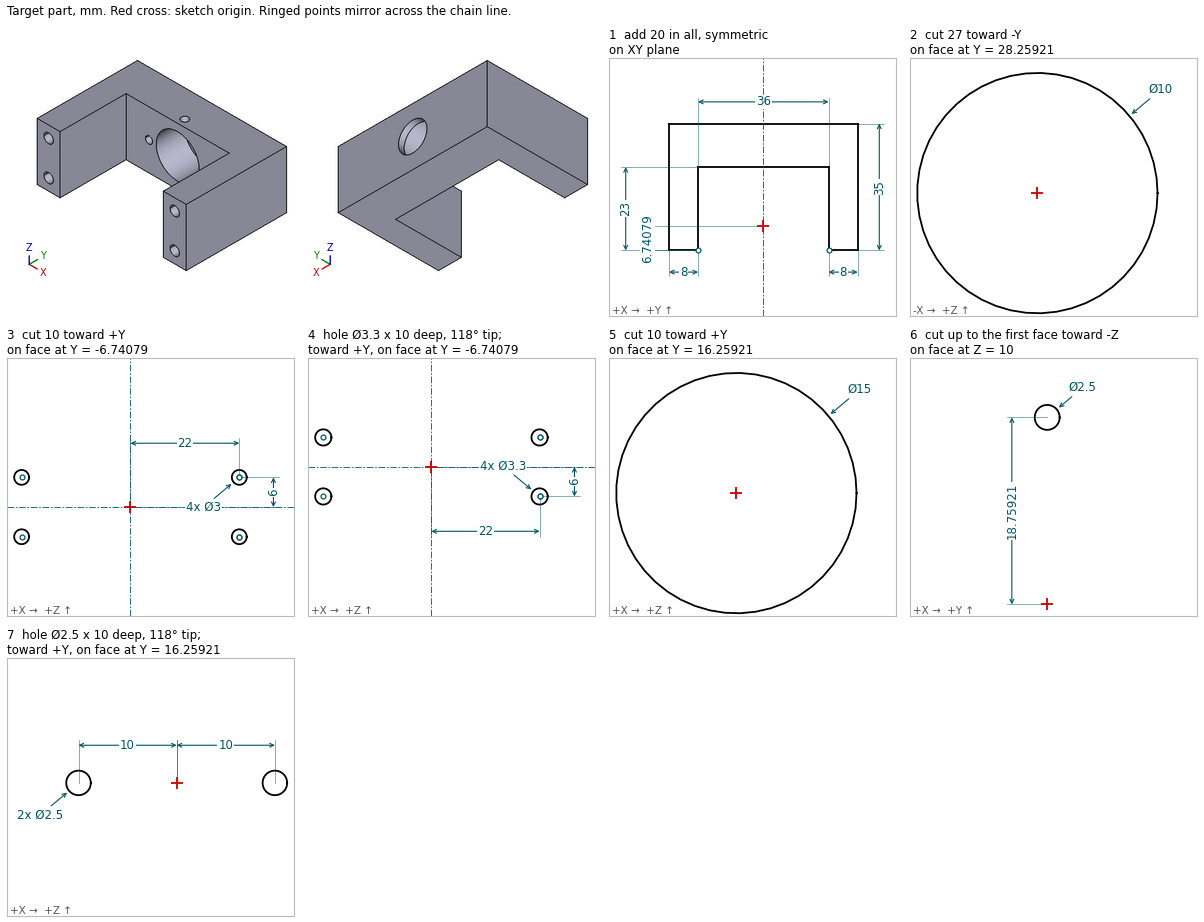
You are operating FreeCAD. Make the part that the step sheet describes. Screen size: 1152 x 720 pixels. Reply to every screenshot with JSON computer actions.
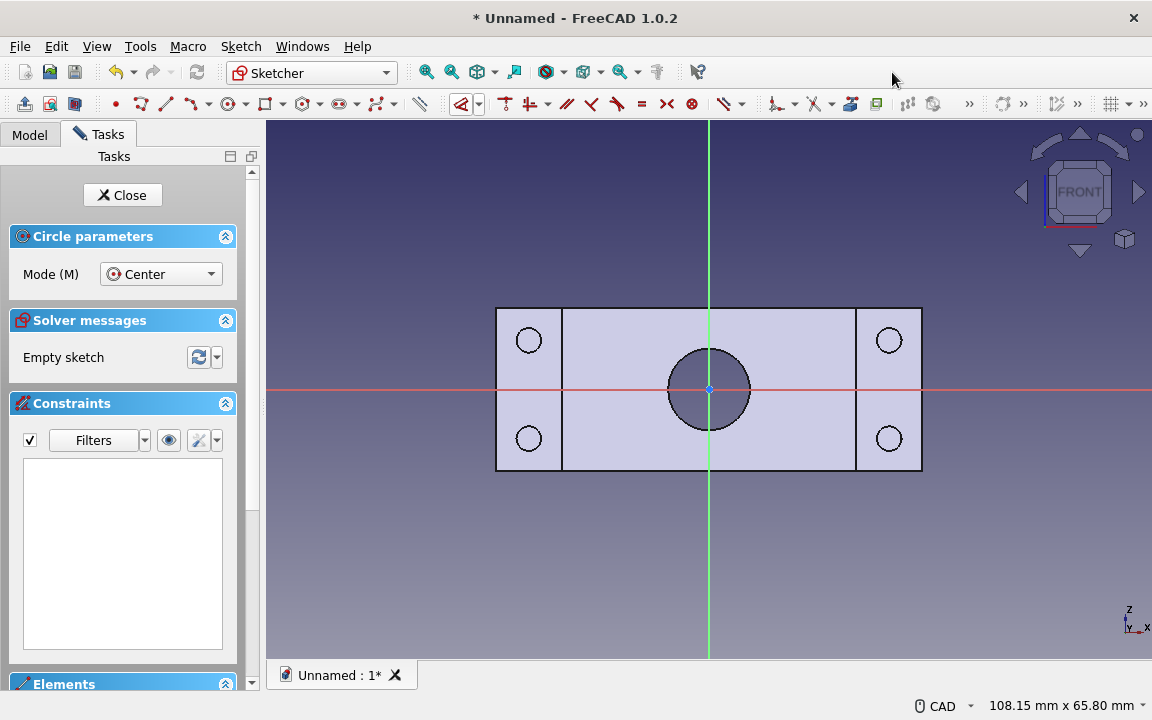
{"action": "scroll", "coordinate": [889, 439], "scroll_direction": "up", "scroll_amount": 3}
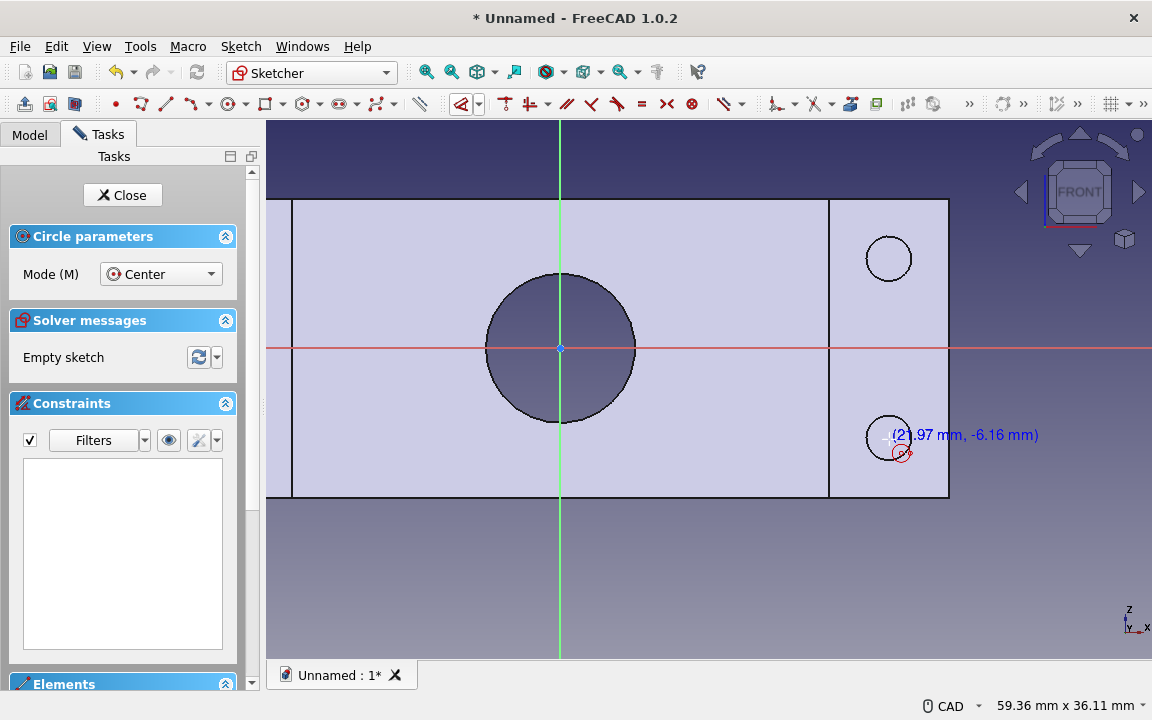
{"action": "left_click", "coordinate": [889, 438]}
{"action": "left_click", "coordinate": [906, 420]}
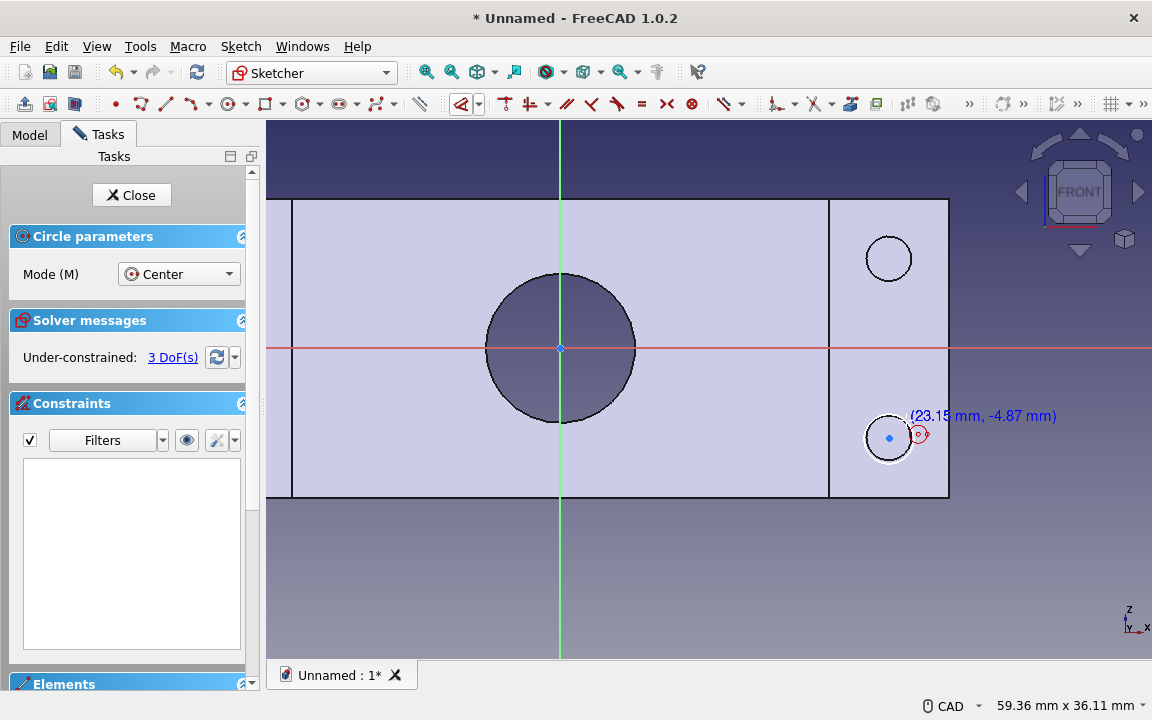
{"action": "left_click", "coordinate": [889, 259]}
{"action": "left_click", "coordinate": [906, 241]}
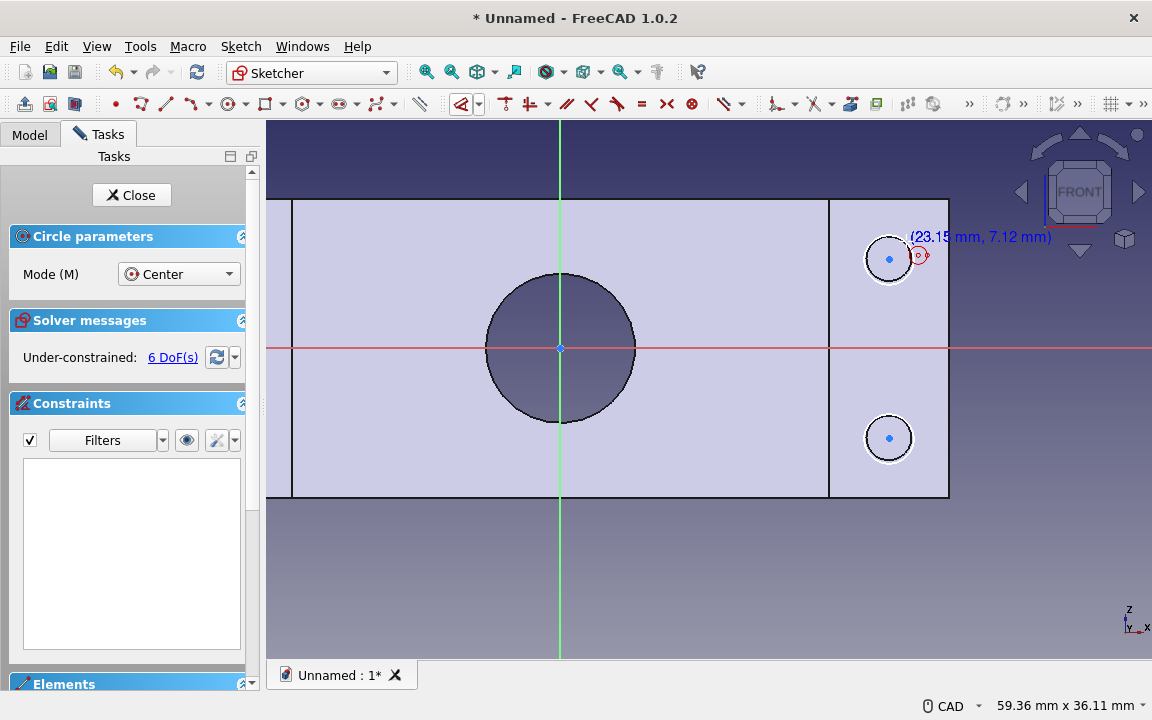
{"action": "scroll", "coordinate": [803, 473], "scroll_direction": "down", "scroll_amount": 2}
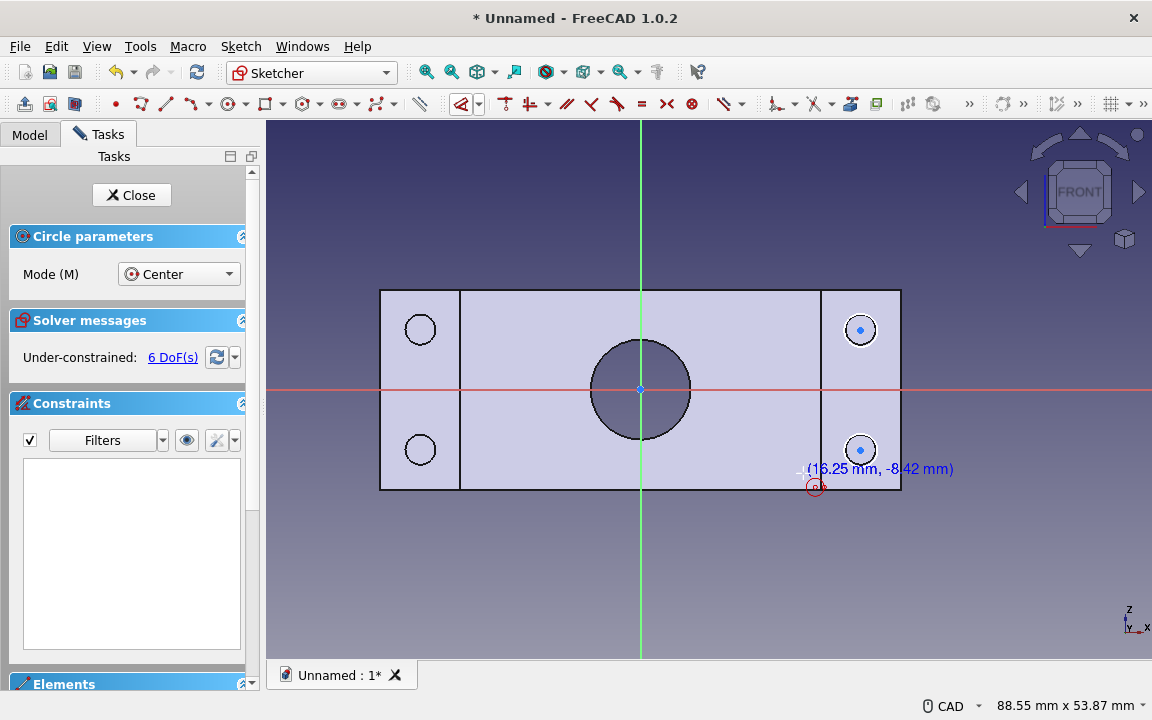
{"action": "scroll", "coordinate": [420, 450], "scroll_direction": "up", "scroll_amount": 2}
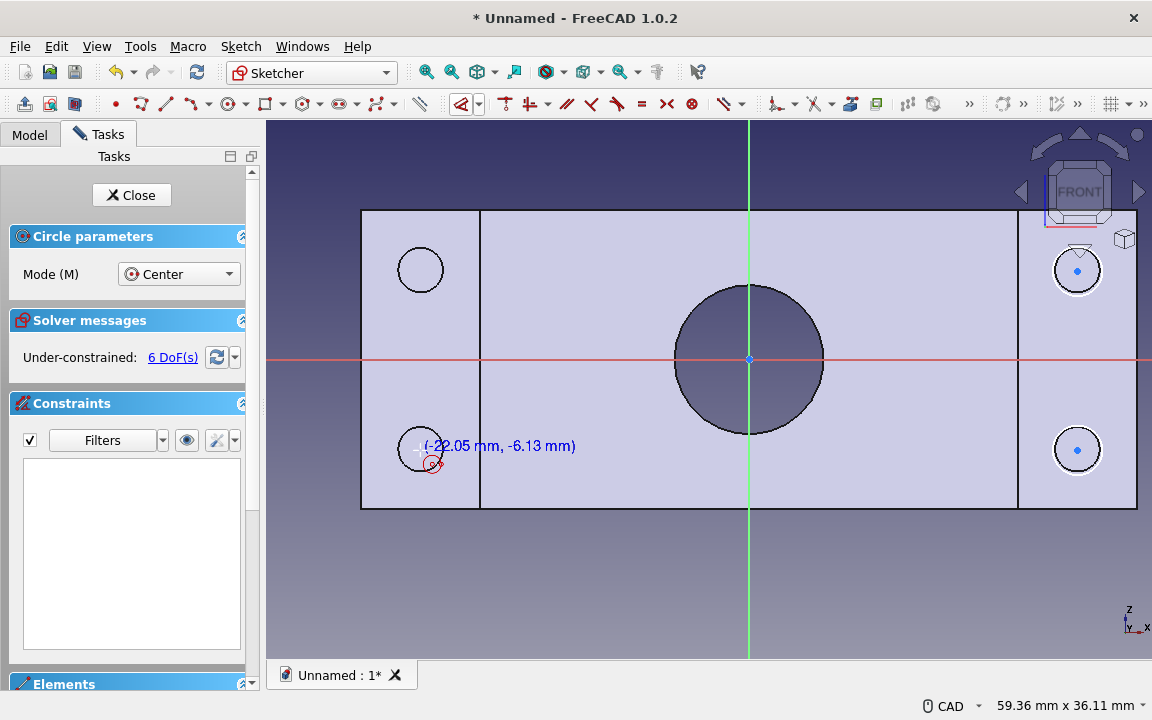
{"action": "left_click", "coordinate": [421, 449]}
{"action": "left_click", "coordinate": [438, 432]}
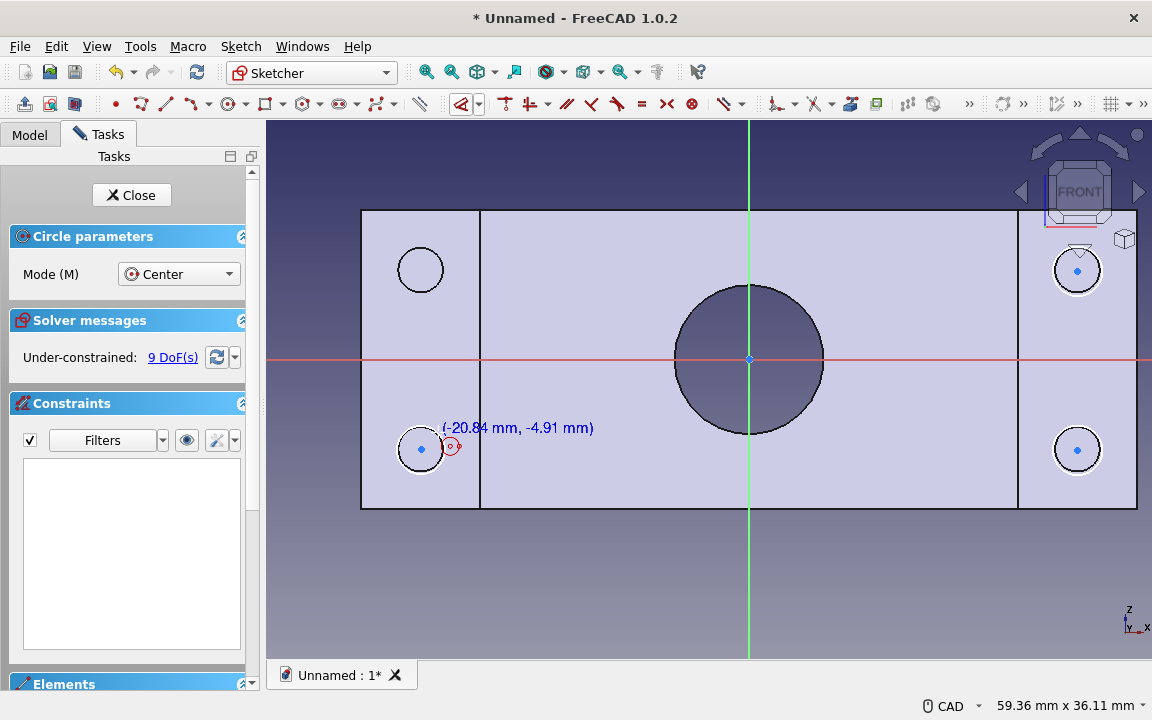
{"action": "left_click", "coordinate": [421, 270]}
{"action": "left_click", "coordinate": [438, 253]}
{"action": "key", "text": "Escape"}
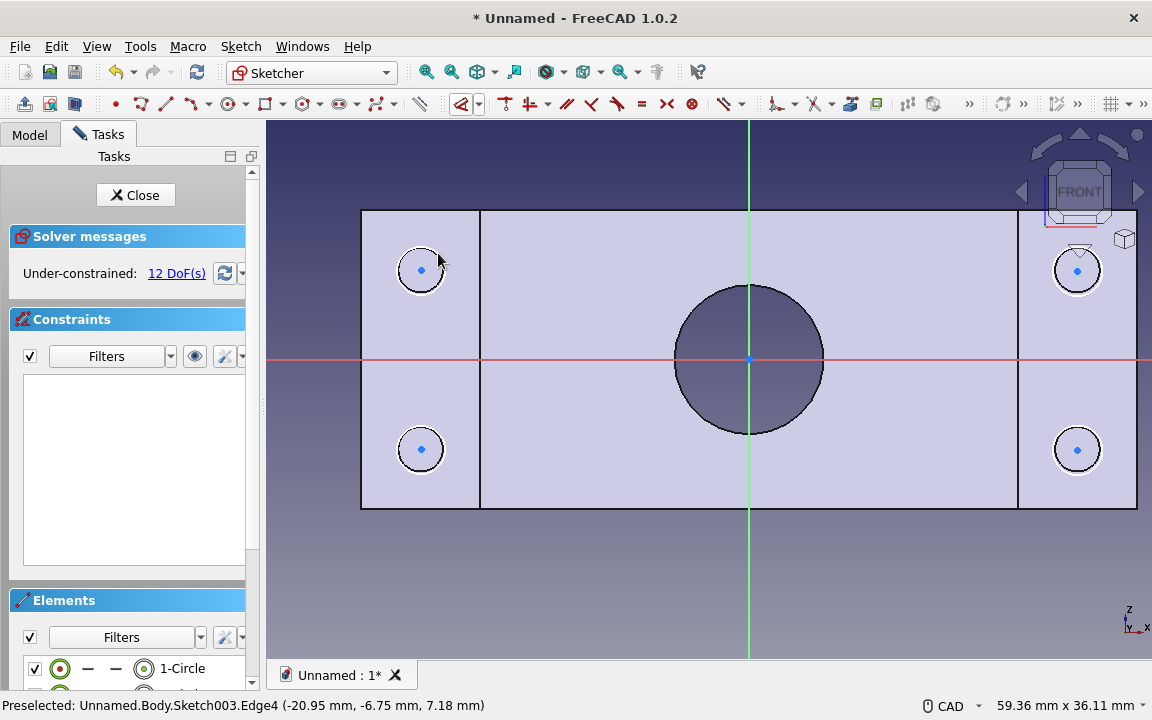
{"action": "scroll", "coordinate": [420, 450], "scroll_direction": "down", "scroll_amount": 2}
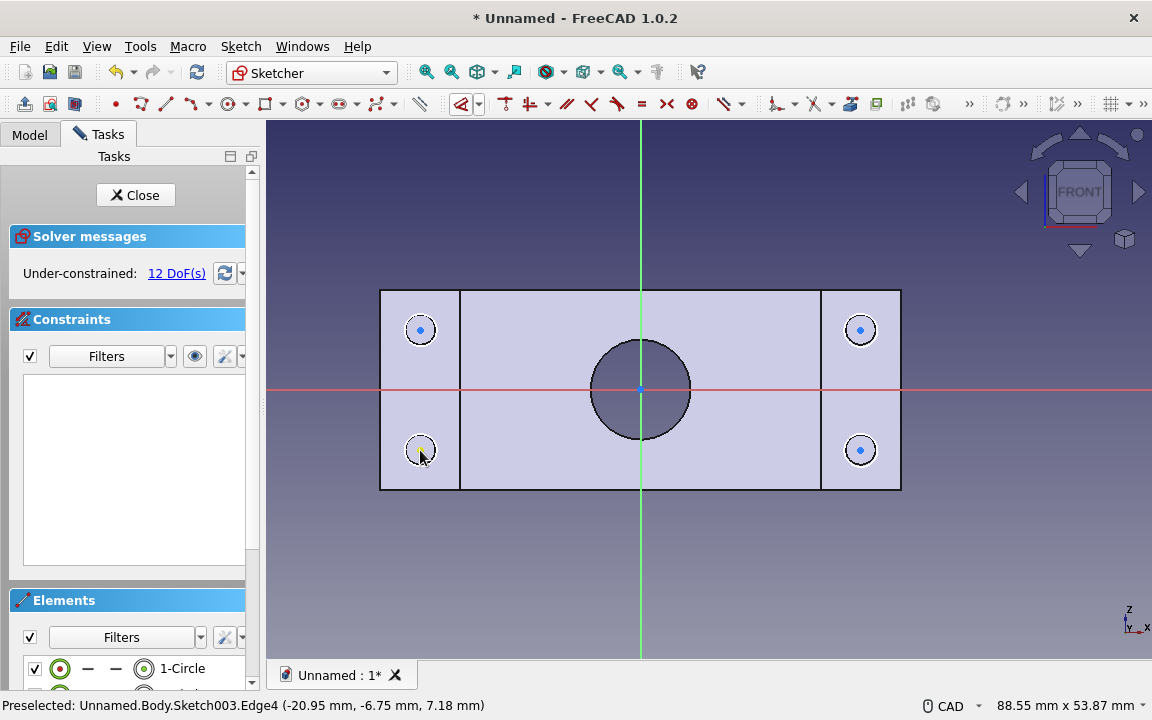
{"action": "left_click", "coordinate": [873, 439]}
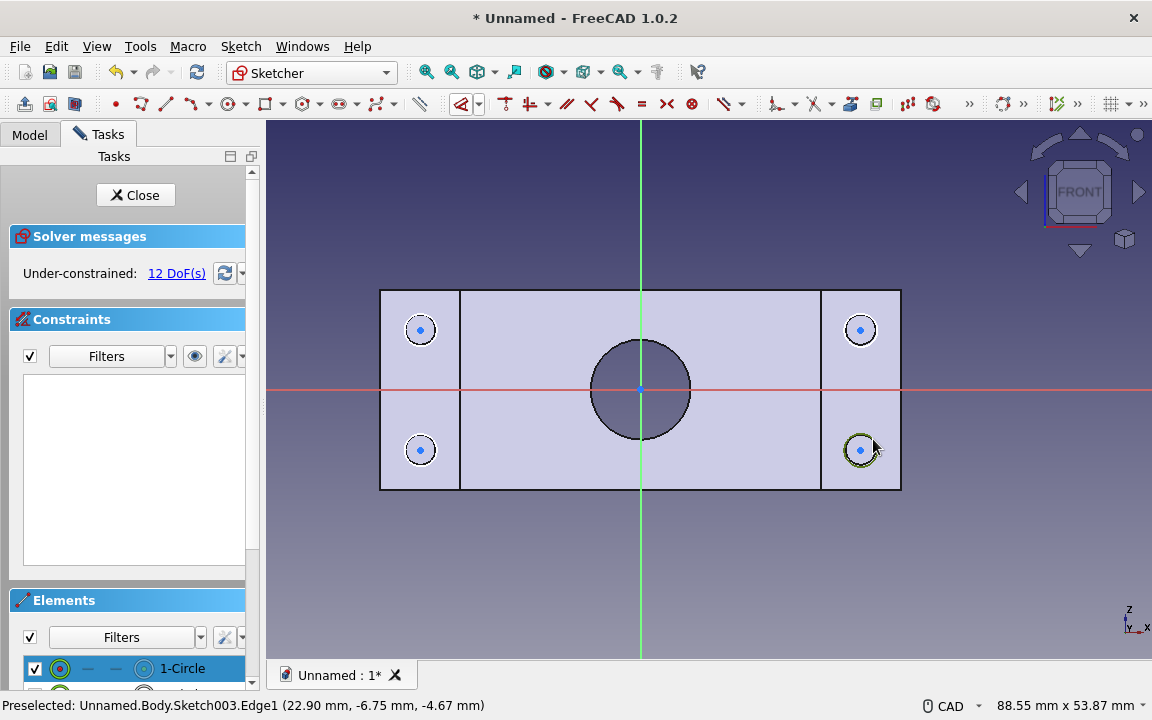
{"action": "left_click", "coordinate": [873, 319]}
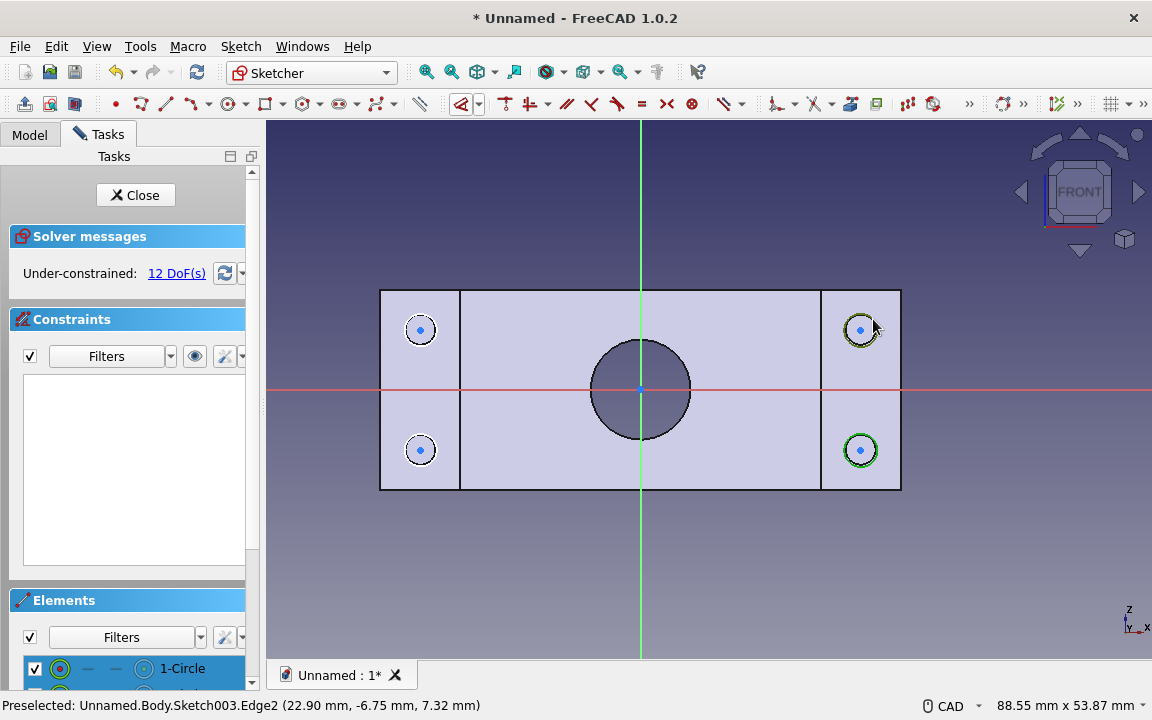
{"action": "left_click", "coordinate": [432, 439]}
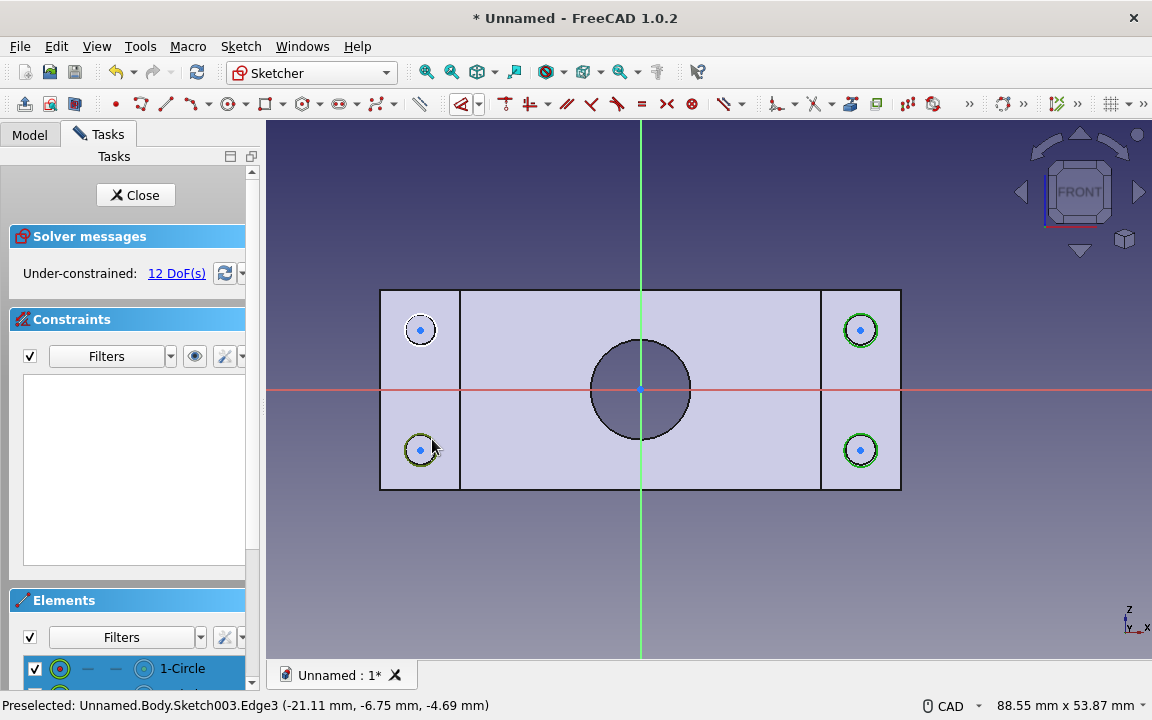
{"action": "left_click", "coordinate": [432, 319]}